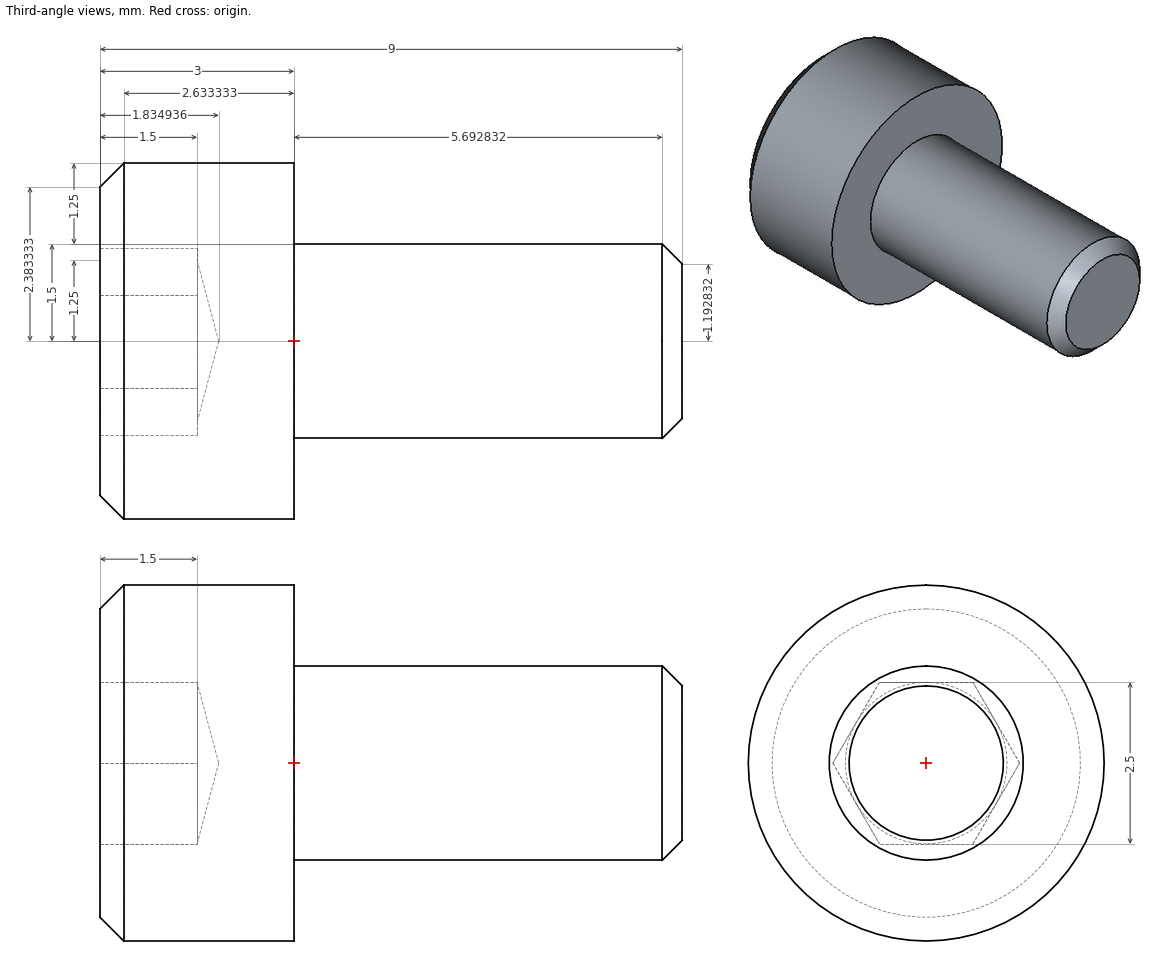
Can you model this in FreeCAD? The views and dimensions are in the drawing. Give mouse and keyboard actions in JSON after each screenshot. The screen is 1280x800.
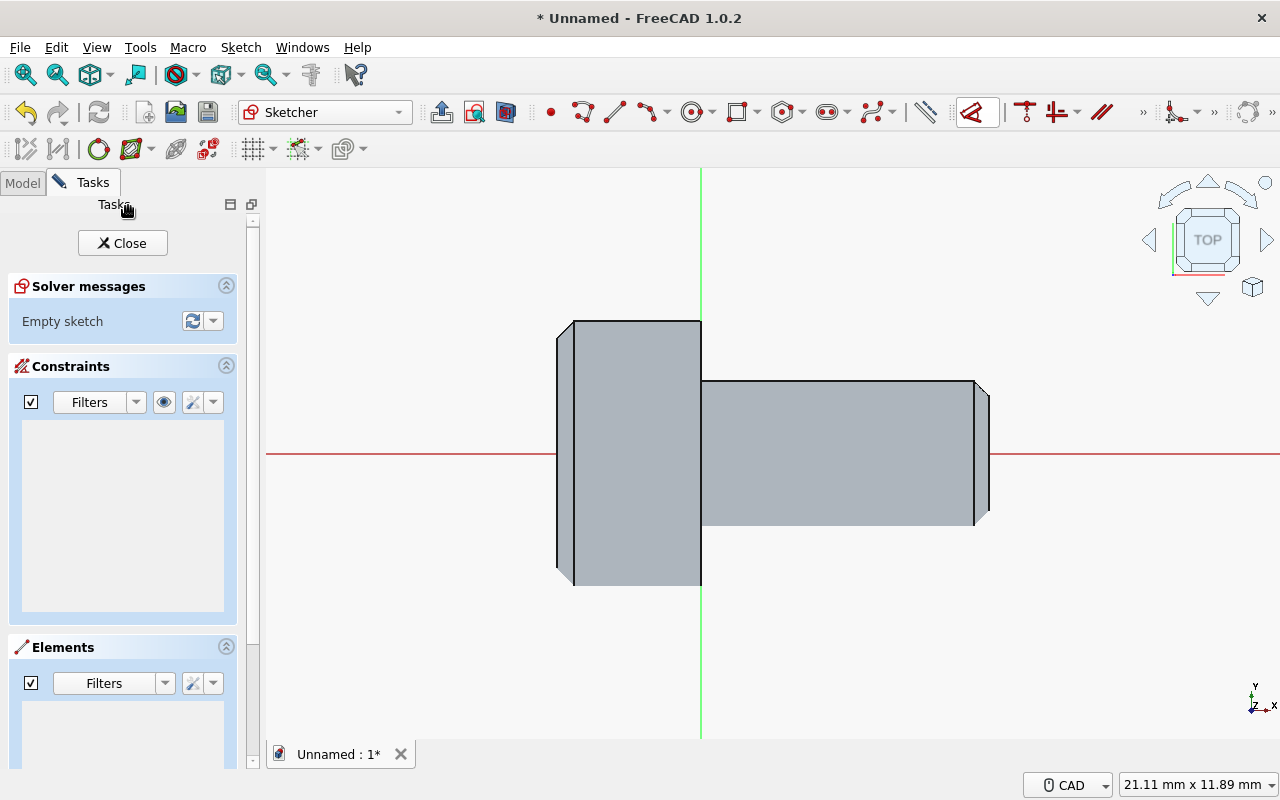
{"action": "left_click", "coordinate": [506, 112]}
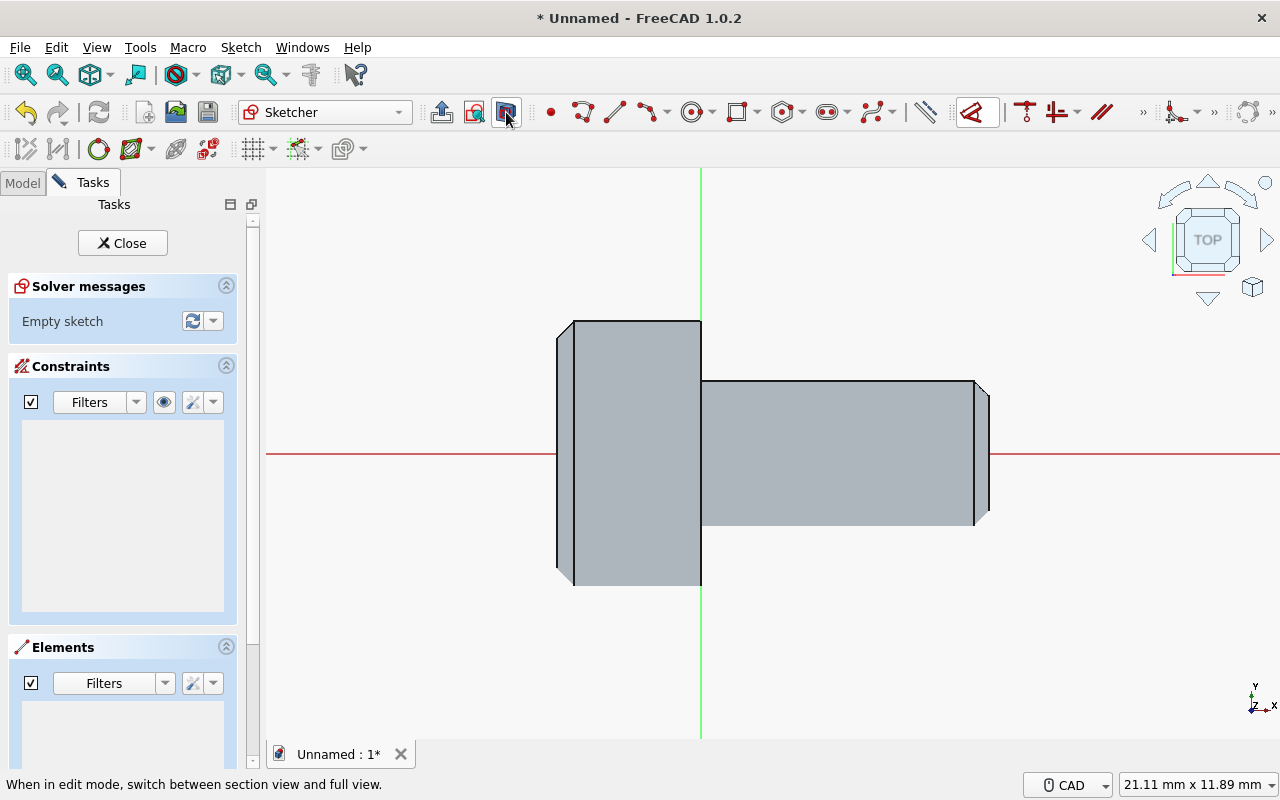
{"action": "scroll", "coordinate": [604, 414], "scroll_direction": "up", "scroll_amount": 7}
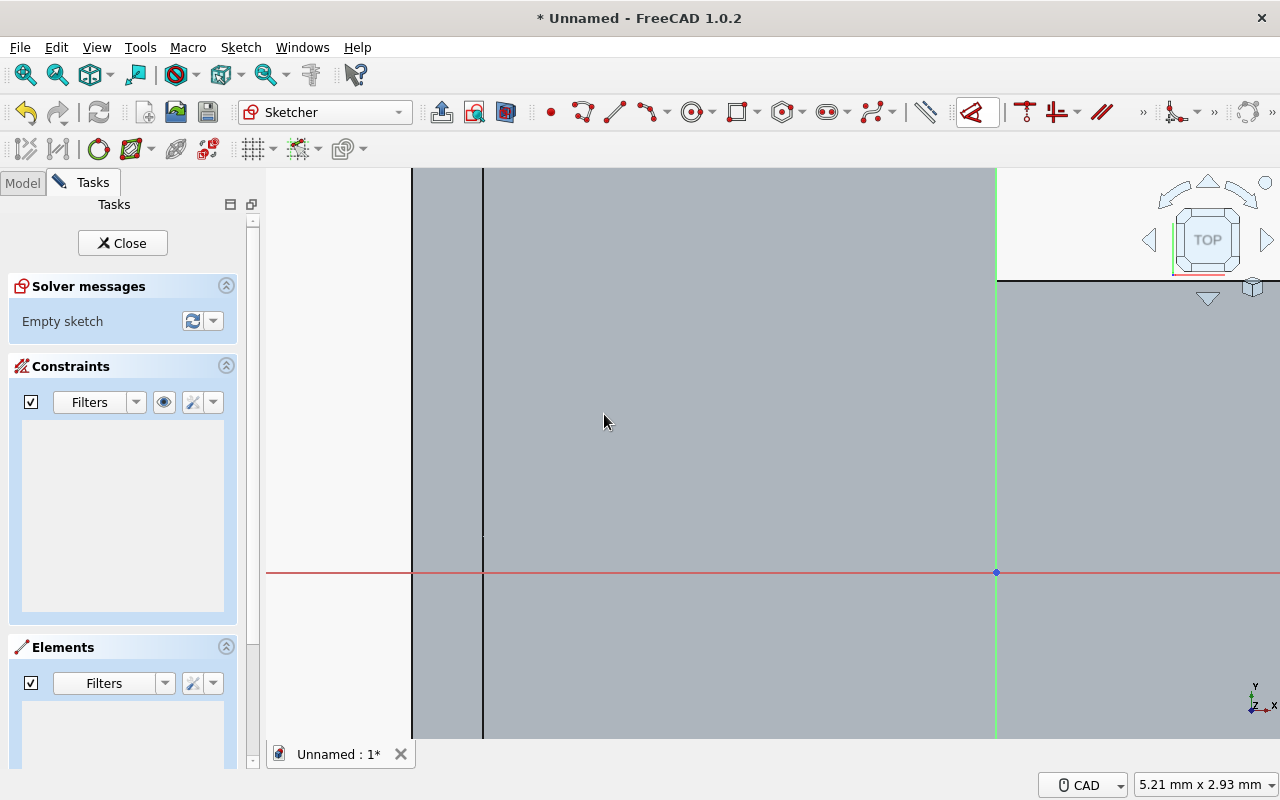
{"action": "key", "text": "g m"}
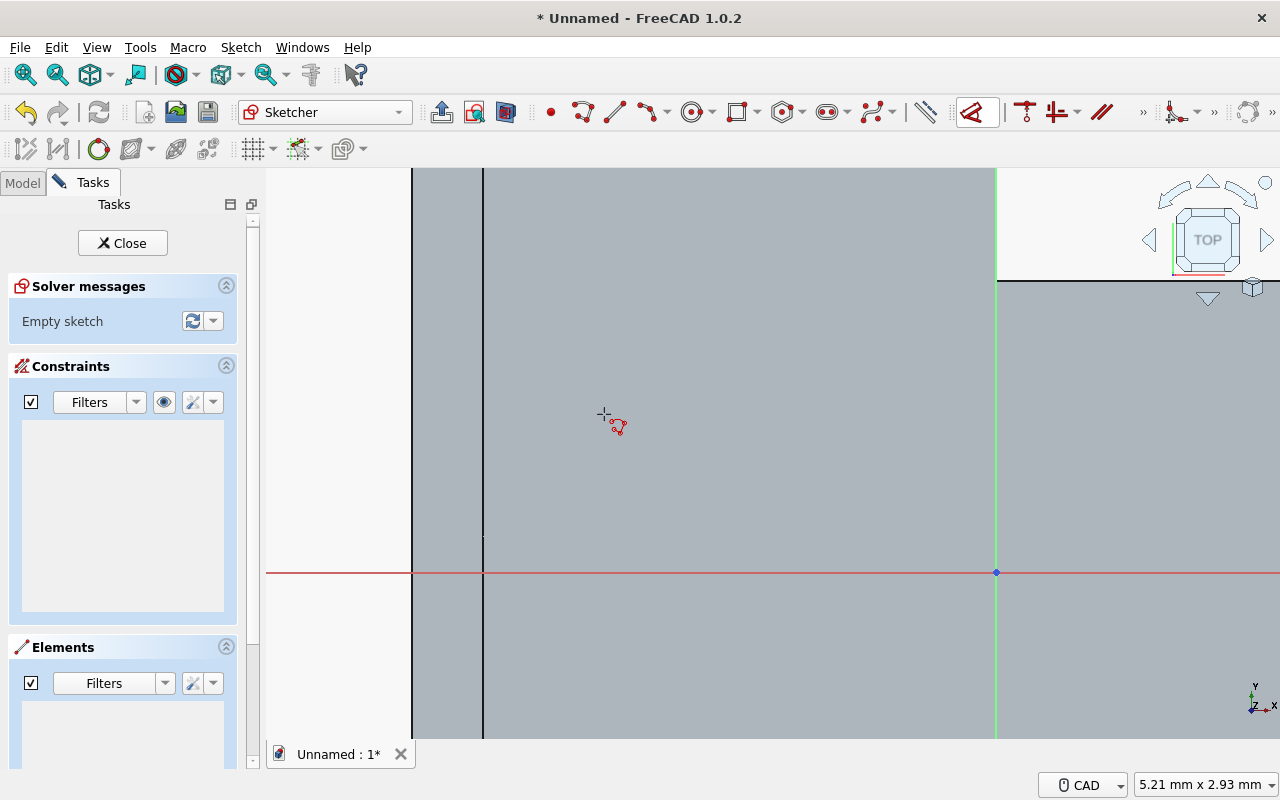
{"action": "left_click", "coordinate": [769, 573]}
{"action": "left_click", "coordinate": [704, 329]}
{"action": "left_click", "coordinate": [412, 329]}
{"action": "left_click", "coordinate": [412, 564]}
{"action": "left_click", "coordinate": [769, 573]}
{"action": "key", "text": "Escape"}
{"action": "key", "text": "Escape"}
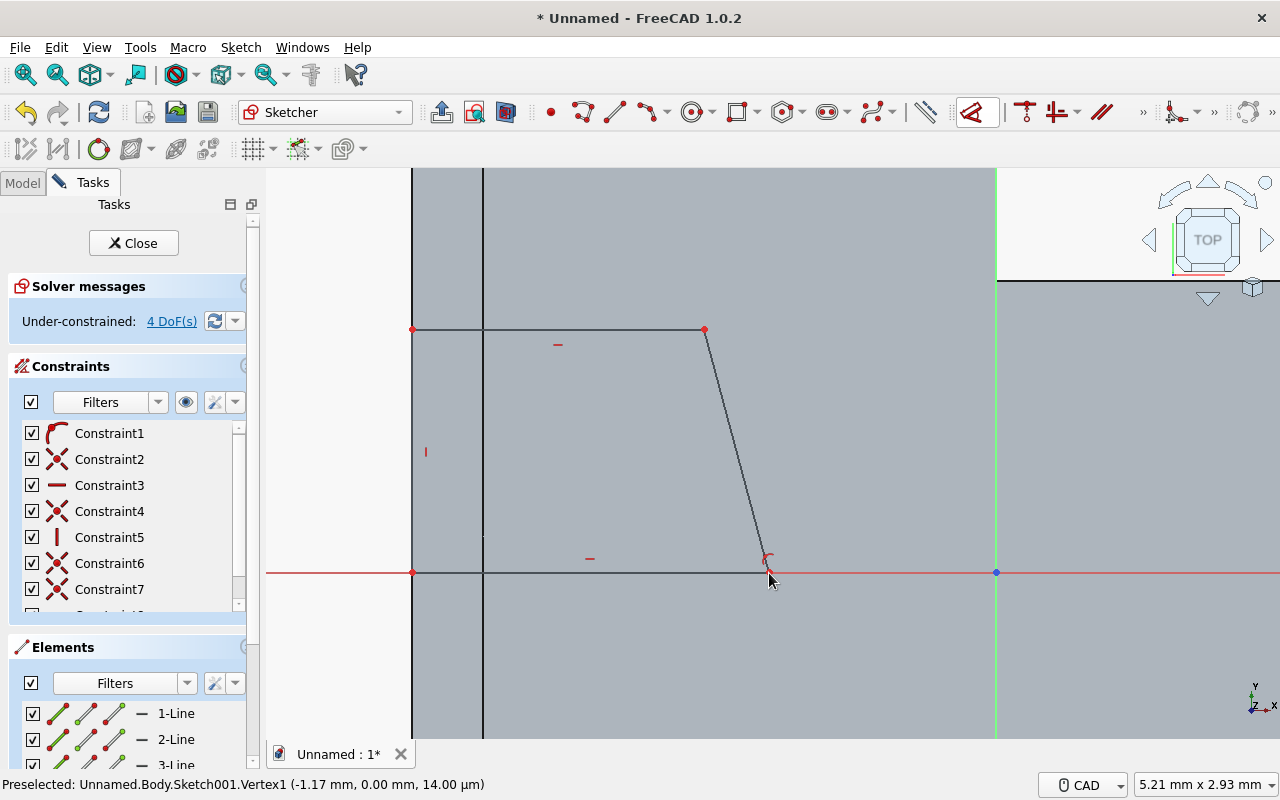
{"action": "left_click", "coordinate": [412, 330]}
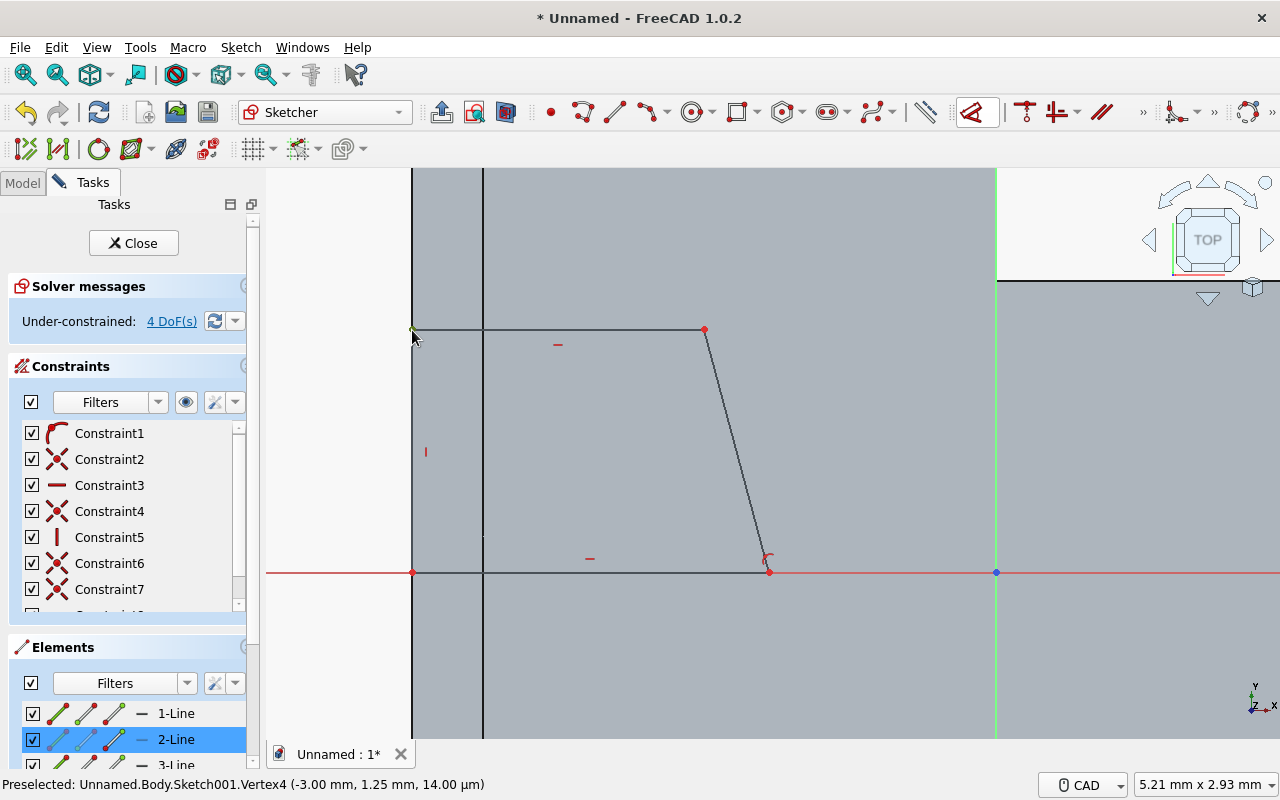
{"action": "left_click", "coordinate": [994, 112]}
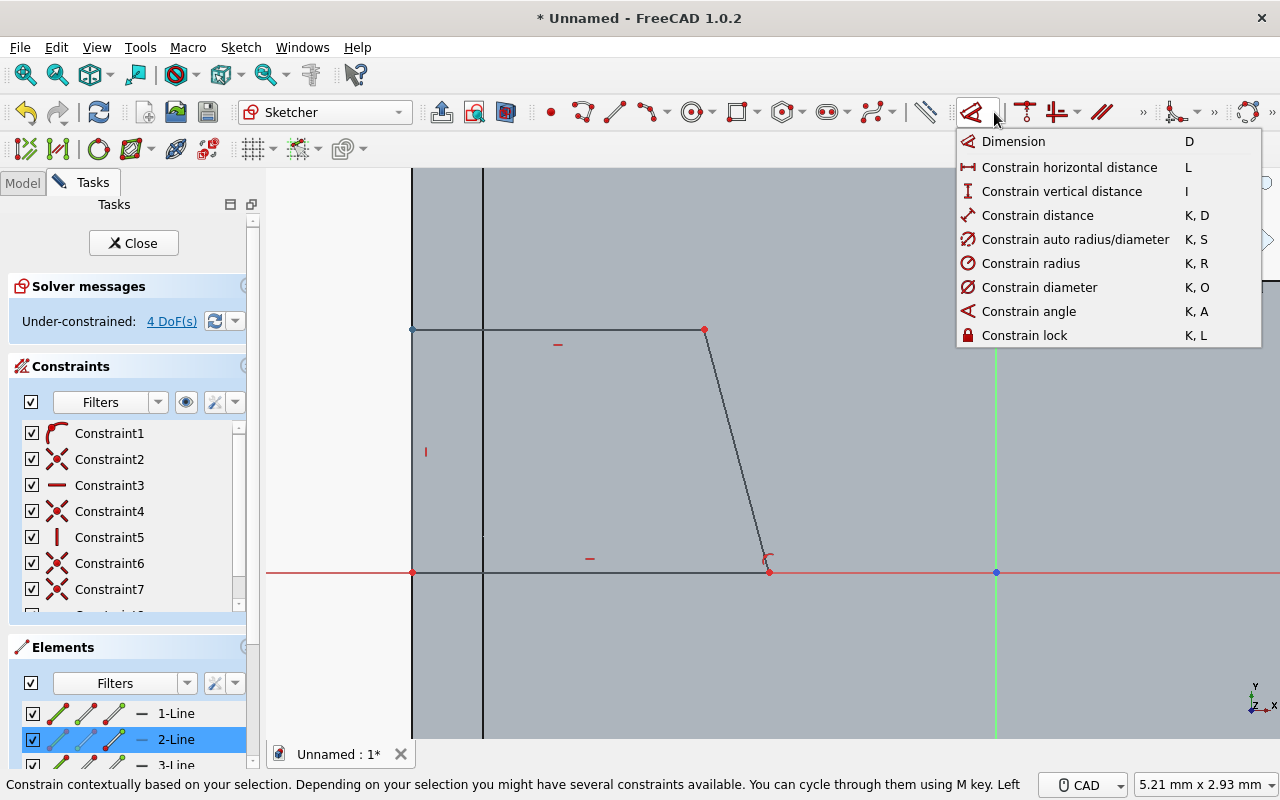
{"action": "left_click", "coordinate": [1109, 167]}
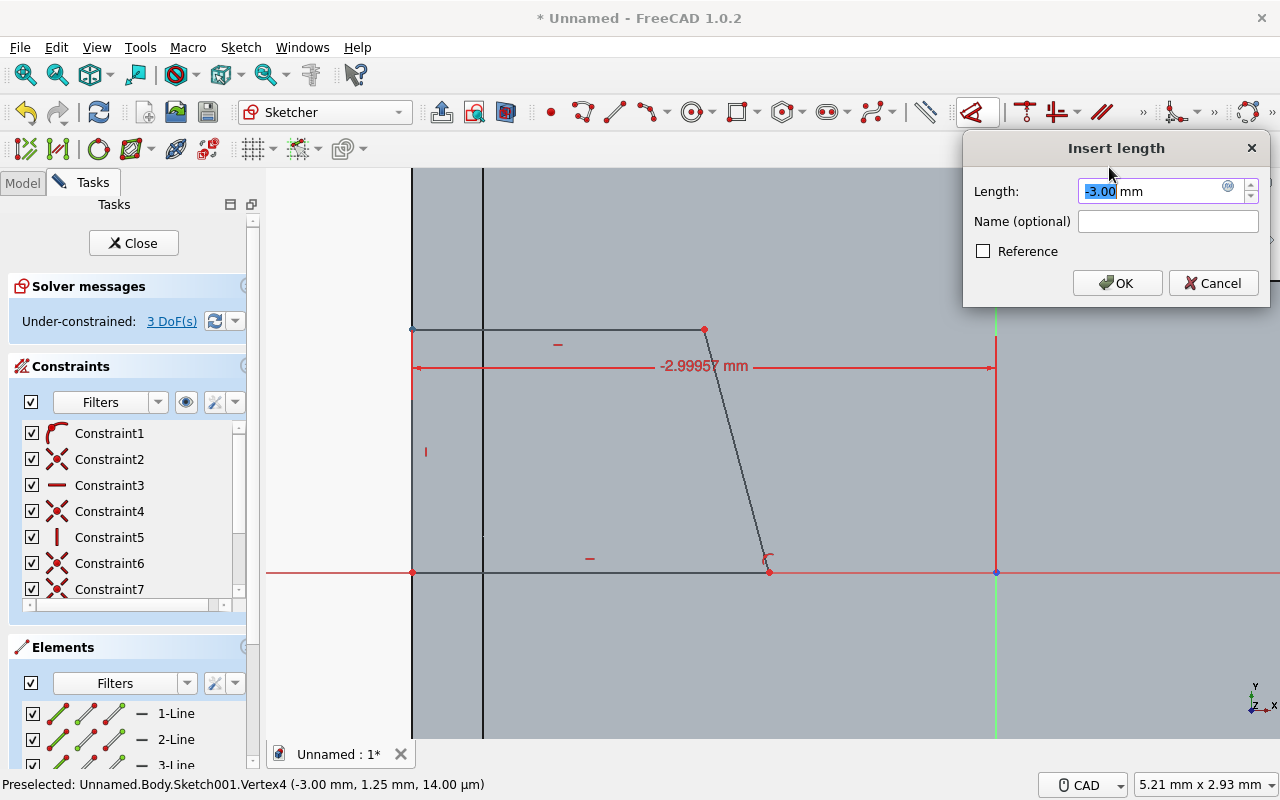
{"action": "type", "text": "-3"}
{"action": "key", "text": "Return"}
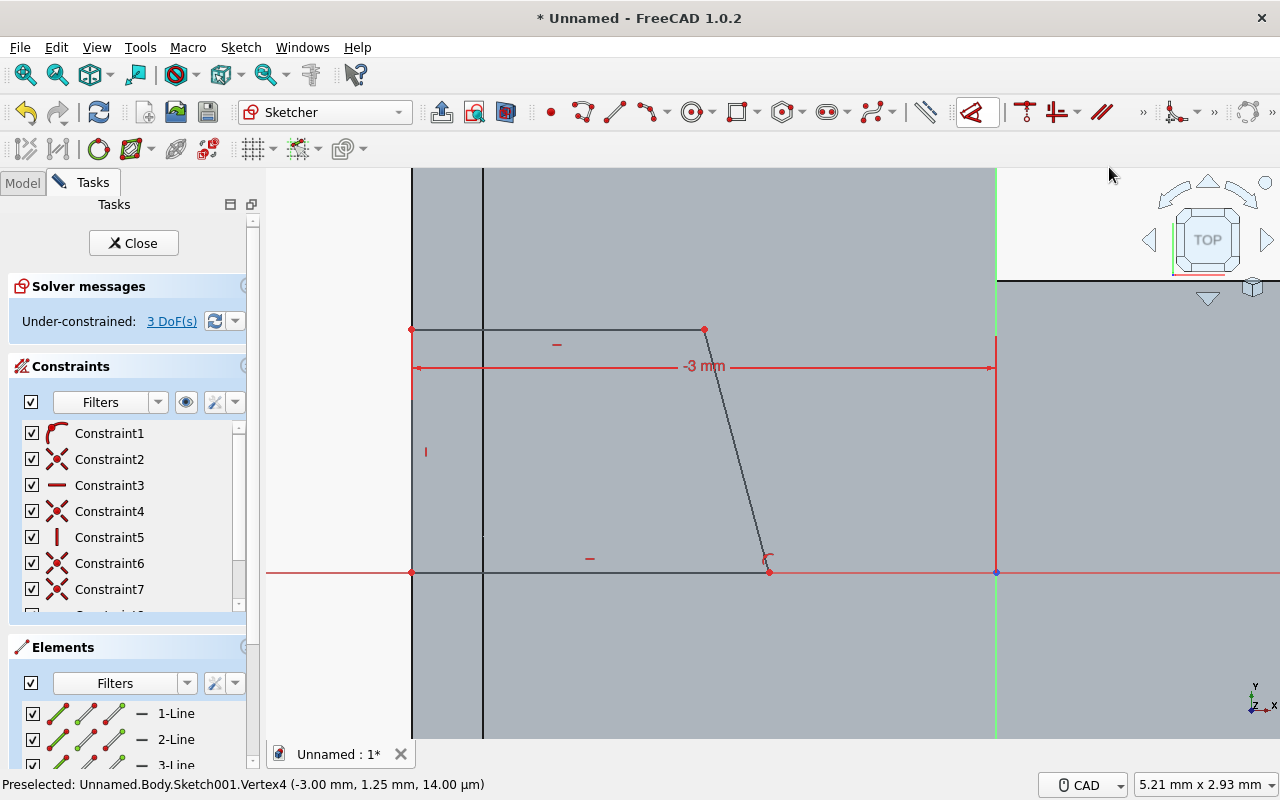
{"action": "left_click", "coordinate": [616, 330]}